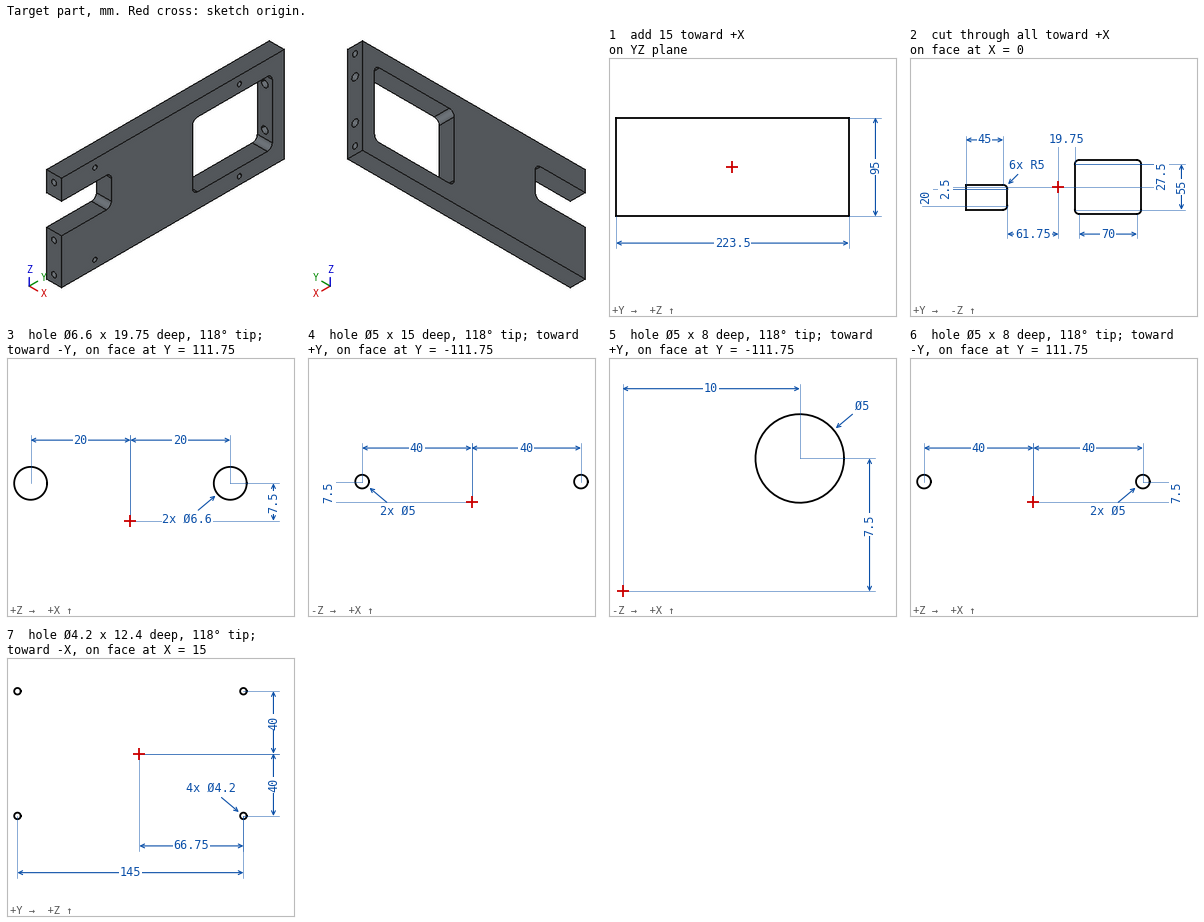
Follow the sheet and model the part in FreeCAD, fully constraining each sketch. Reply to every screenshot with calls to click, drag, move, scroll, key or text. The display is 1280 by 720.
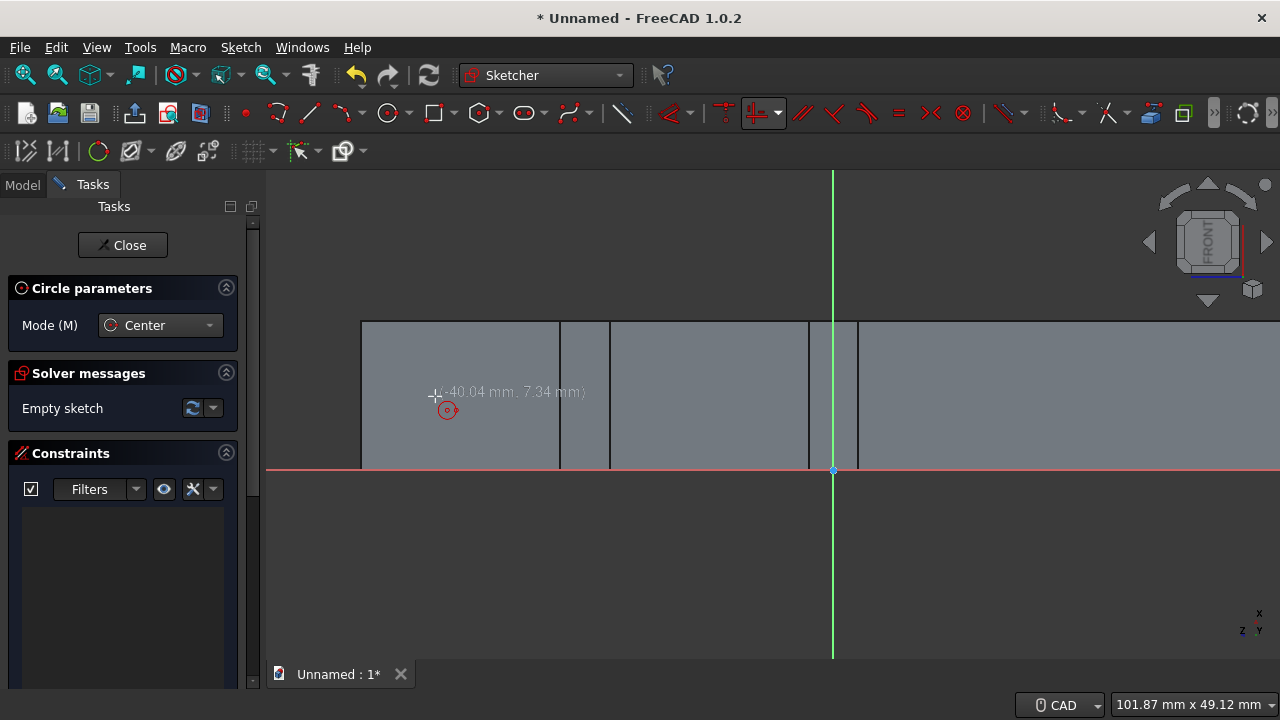
click(435, 396)
move(453, 378)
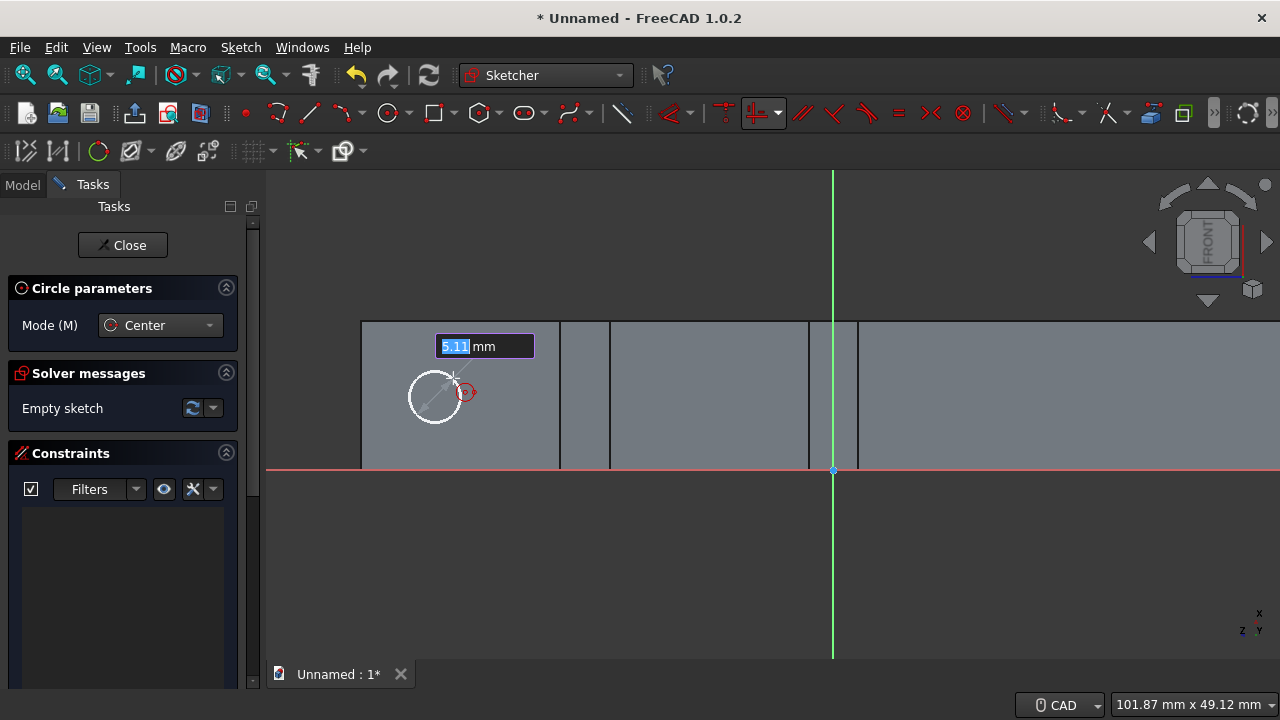
text(5)
key(Return)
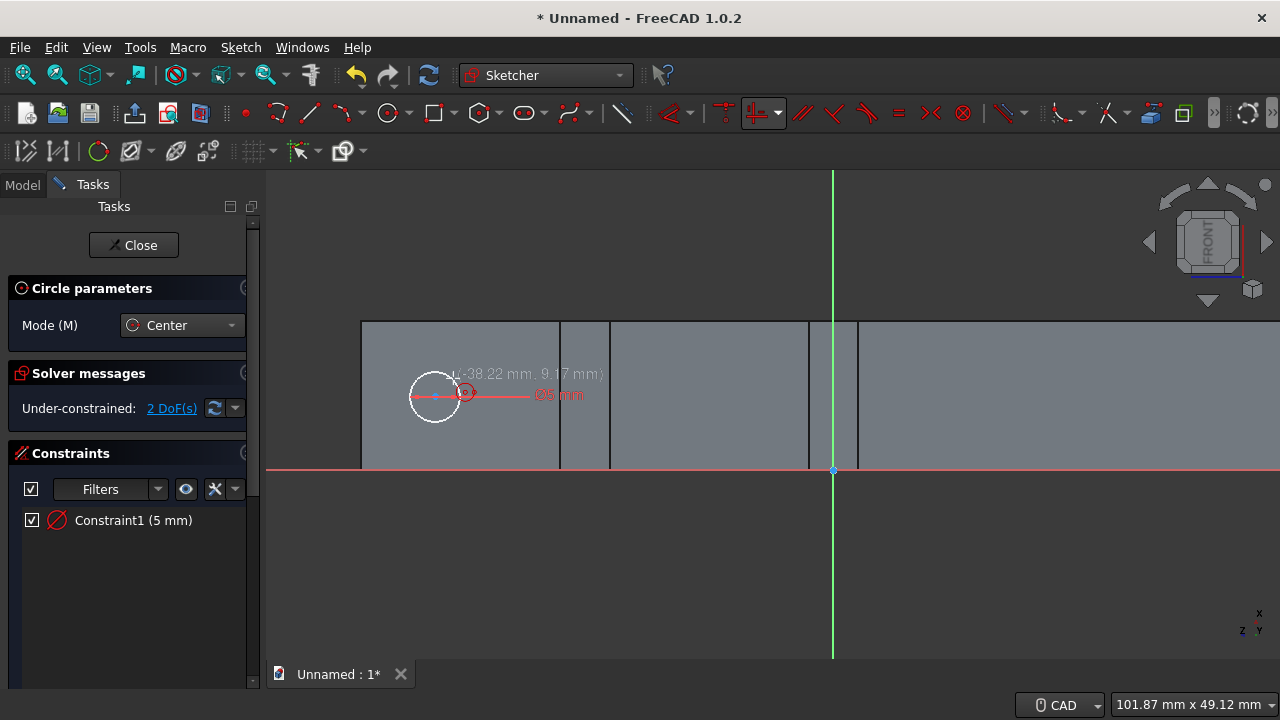
scroll(442, 402, down, 2)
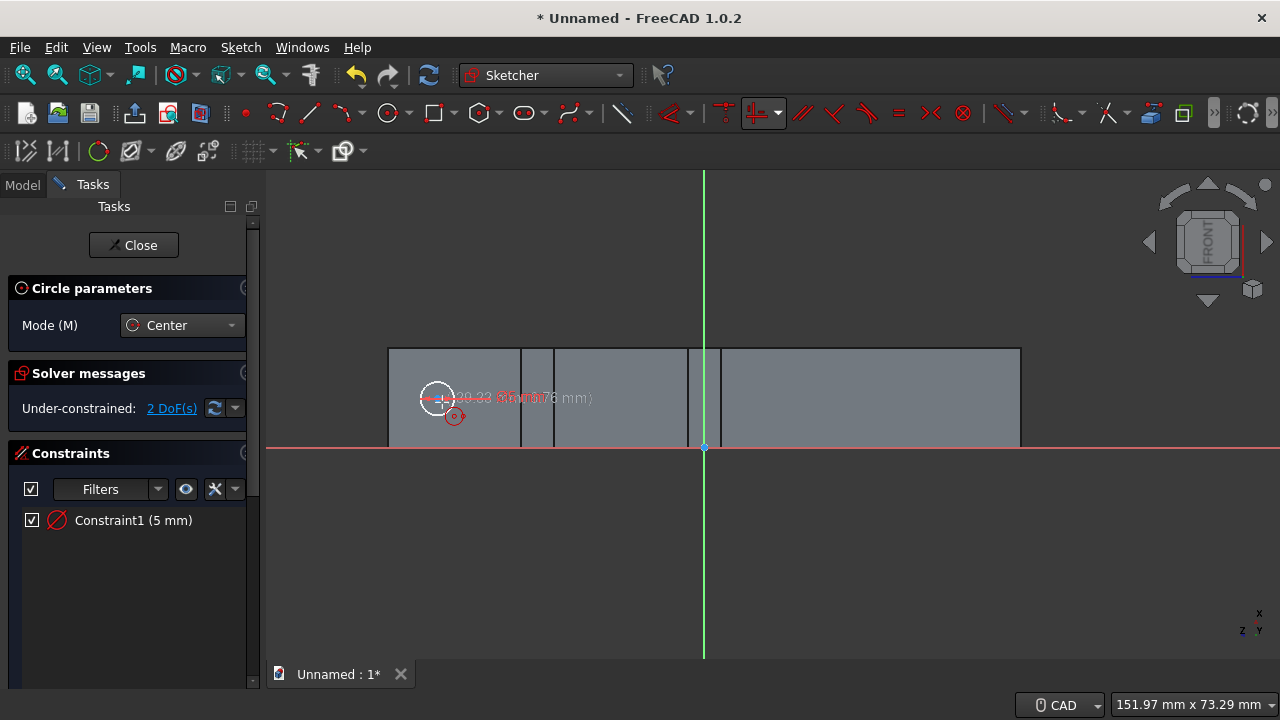
scroll(971, 398, up, 2)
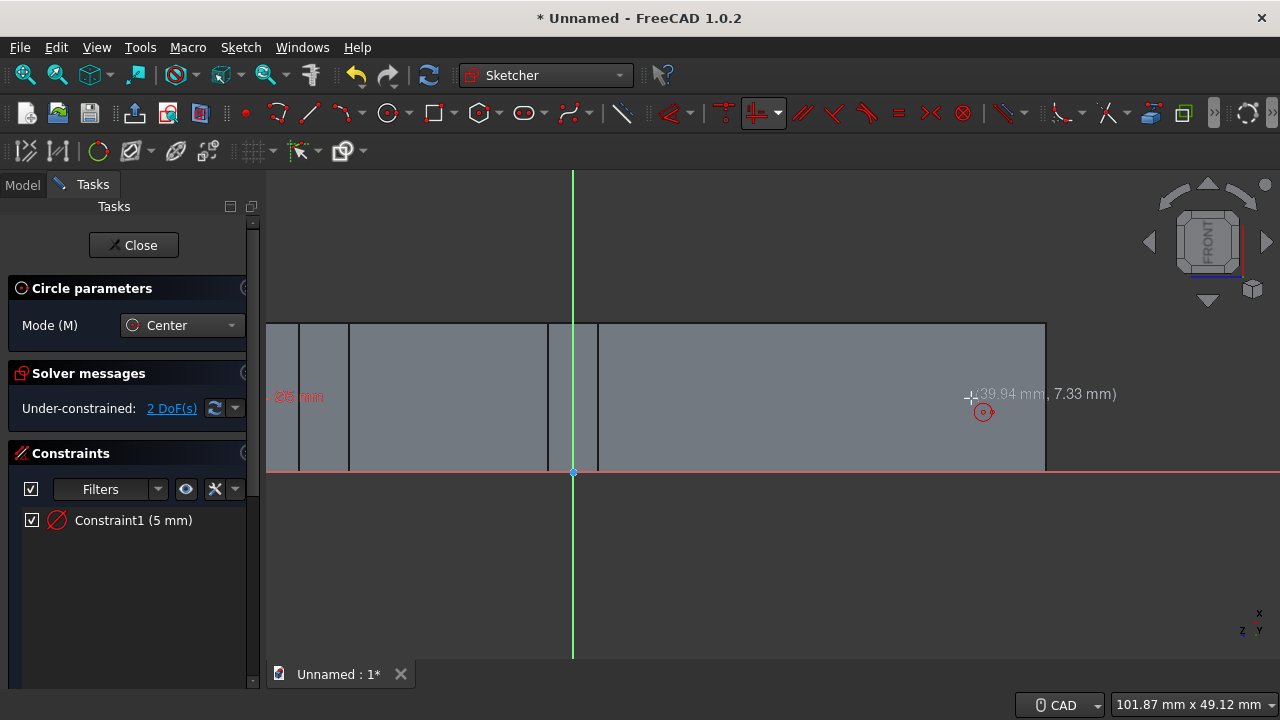
click(971, 398)
move(989, 380)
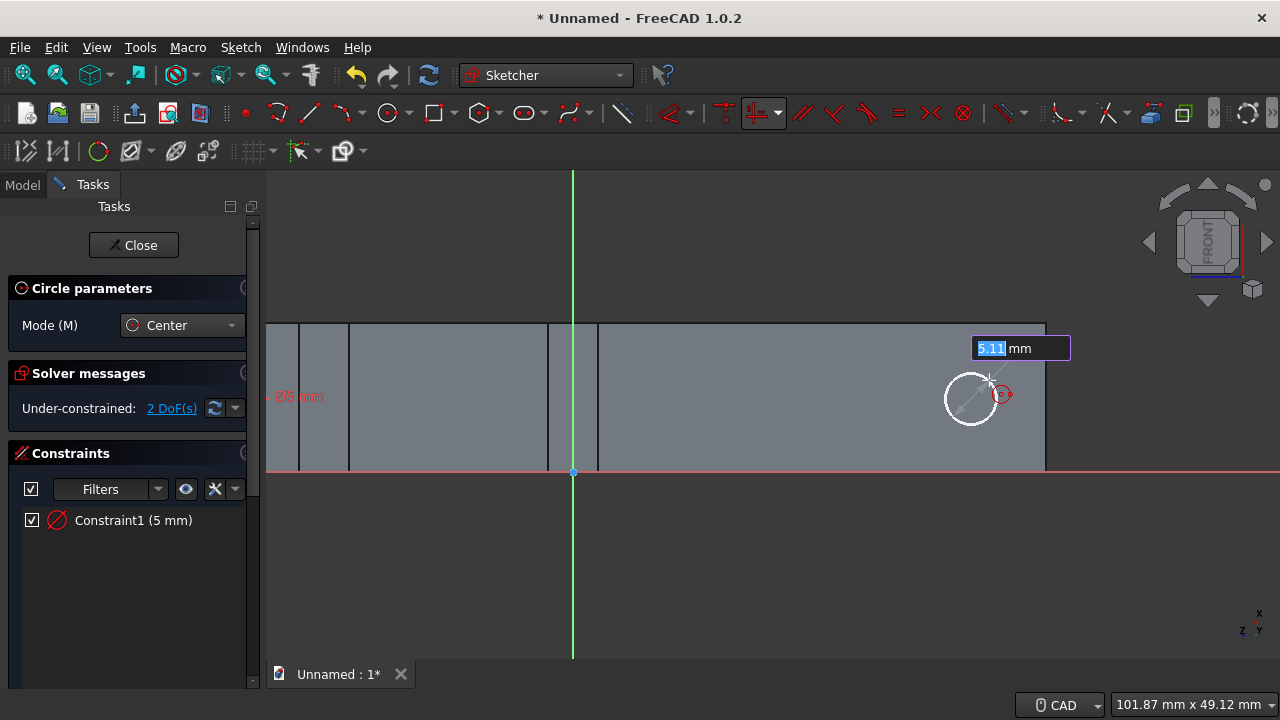
text(5)
key(Return)
key(Escape)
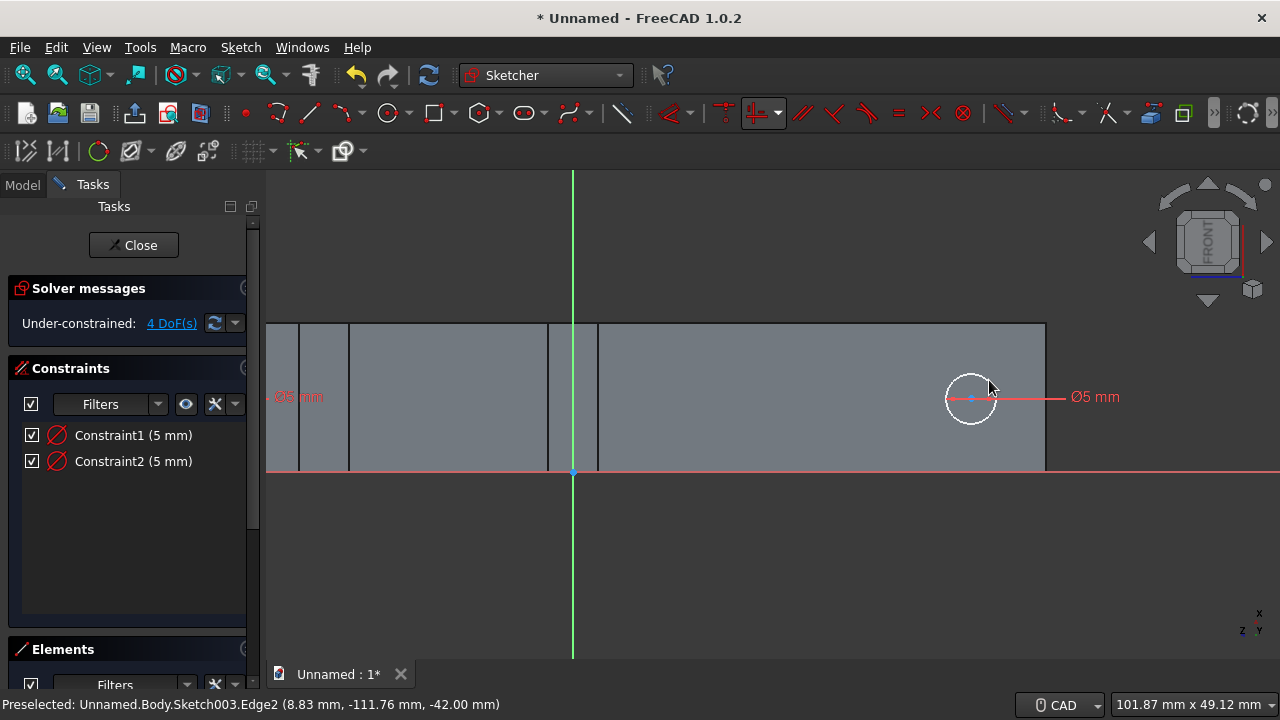
scroll(972, 398, down, 2)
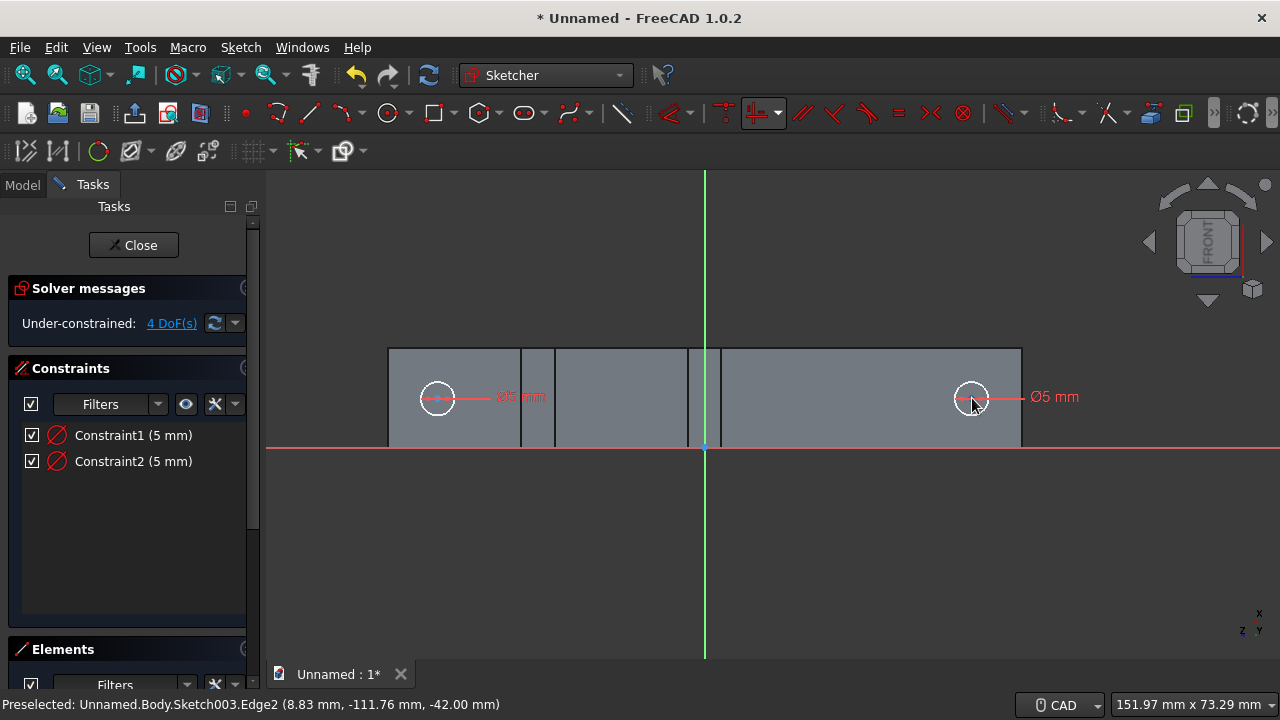
click(438, 399)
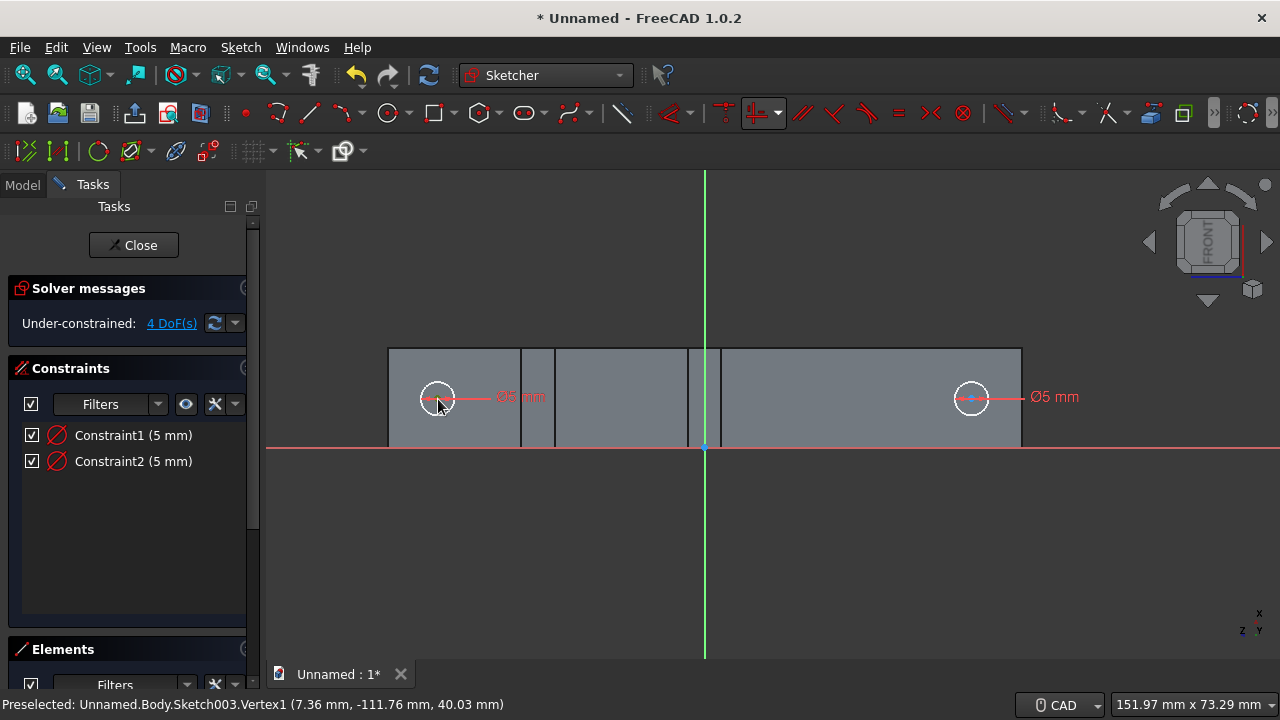
click(972, 399)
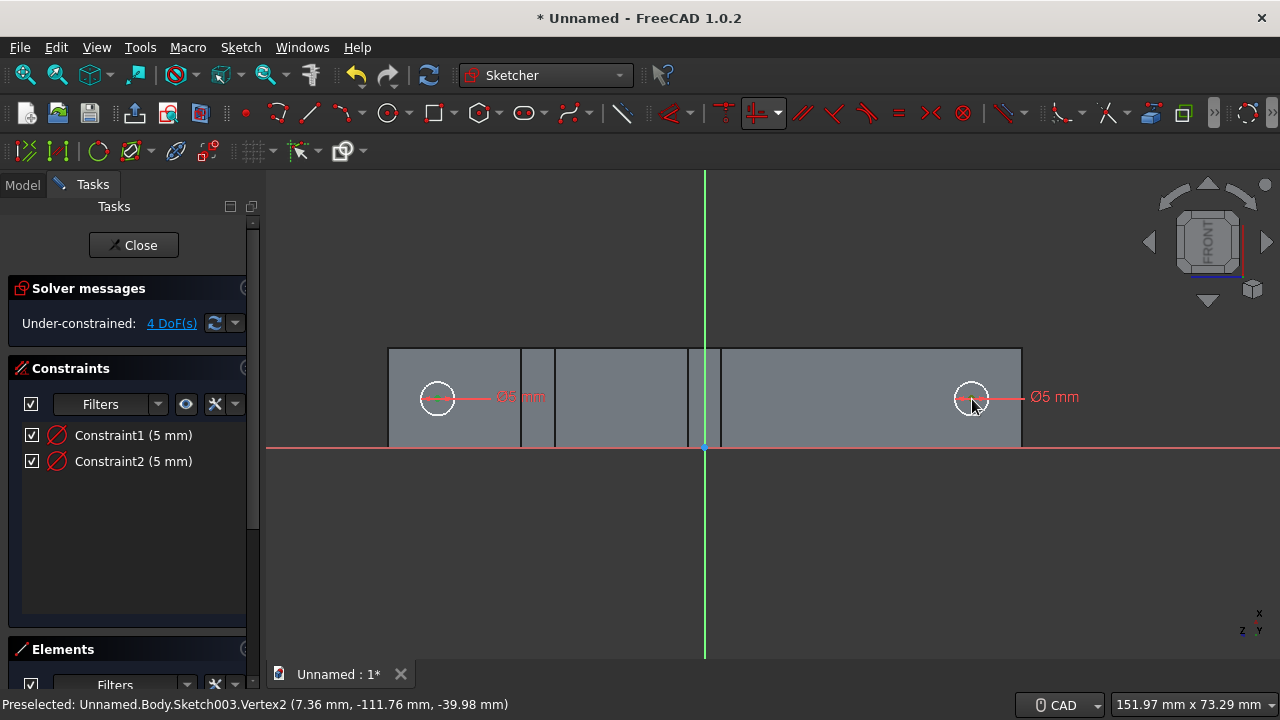
key(h)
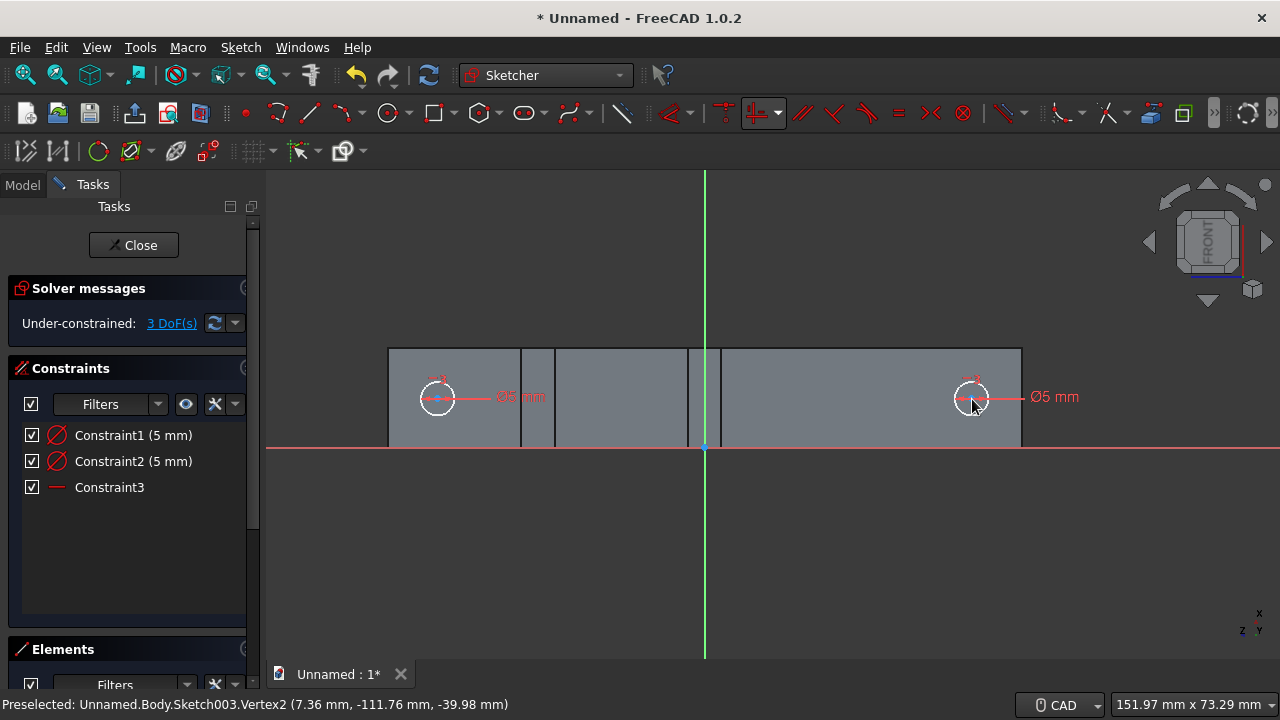
click(670, 114)